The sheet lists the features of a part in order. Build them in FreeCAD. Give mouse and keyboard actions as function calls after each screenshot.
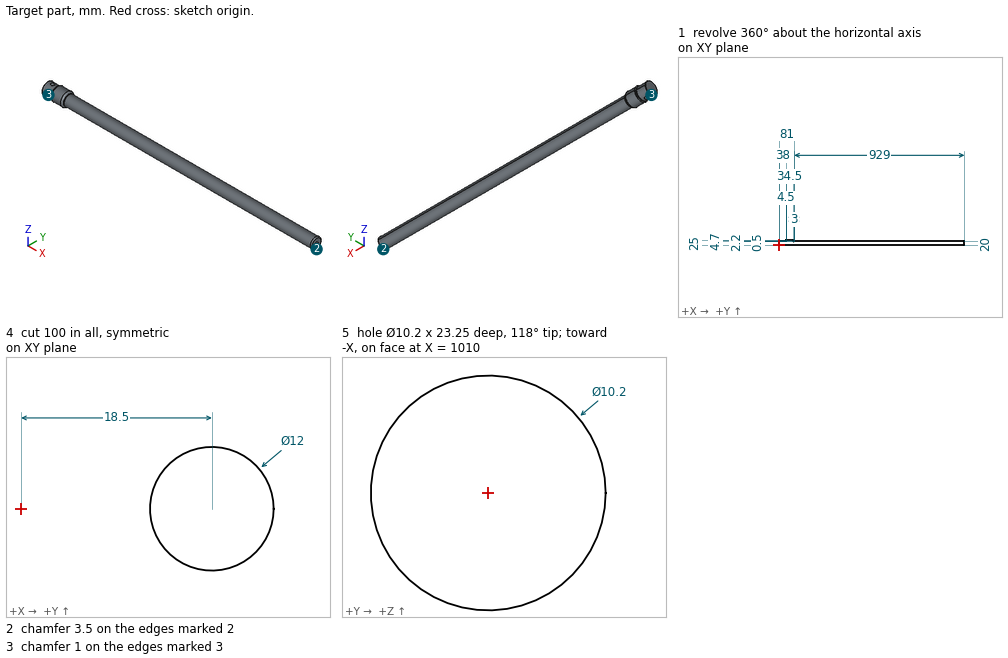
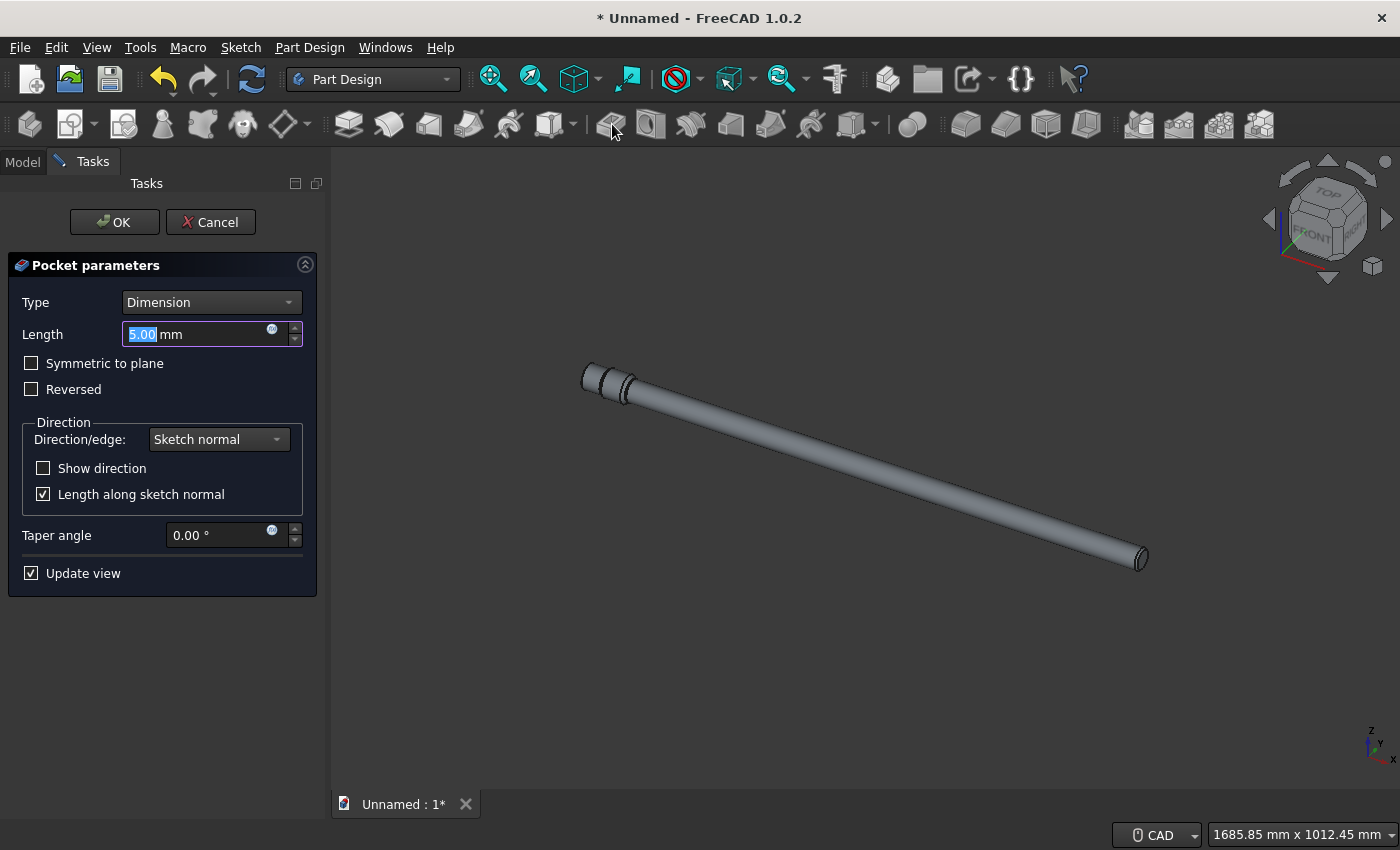
text(100)
key(Tab)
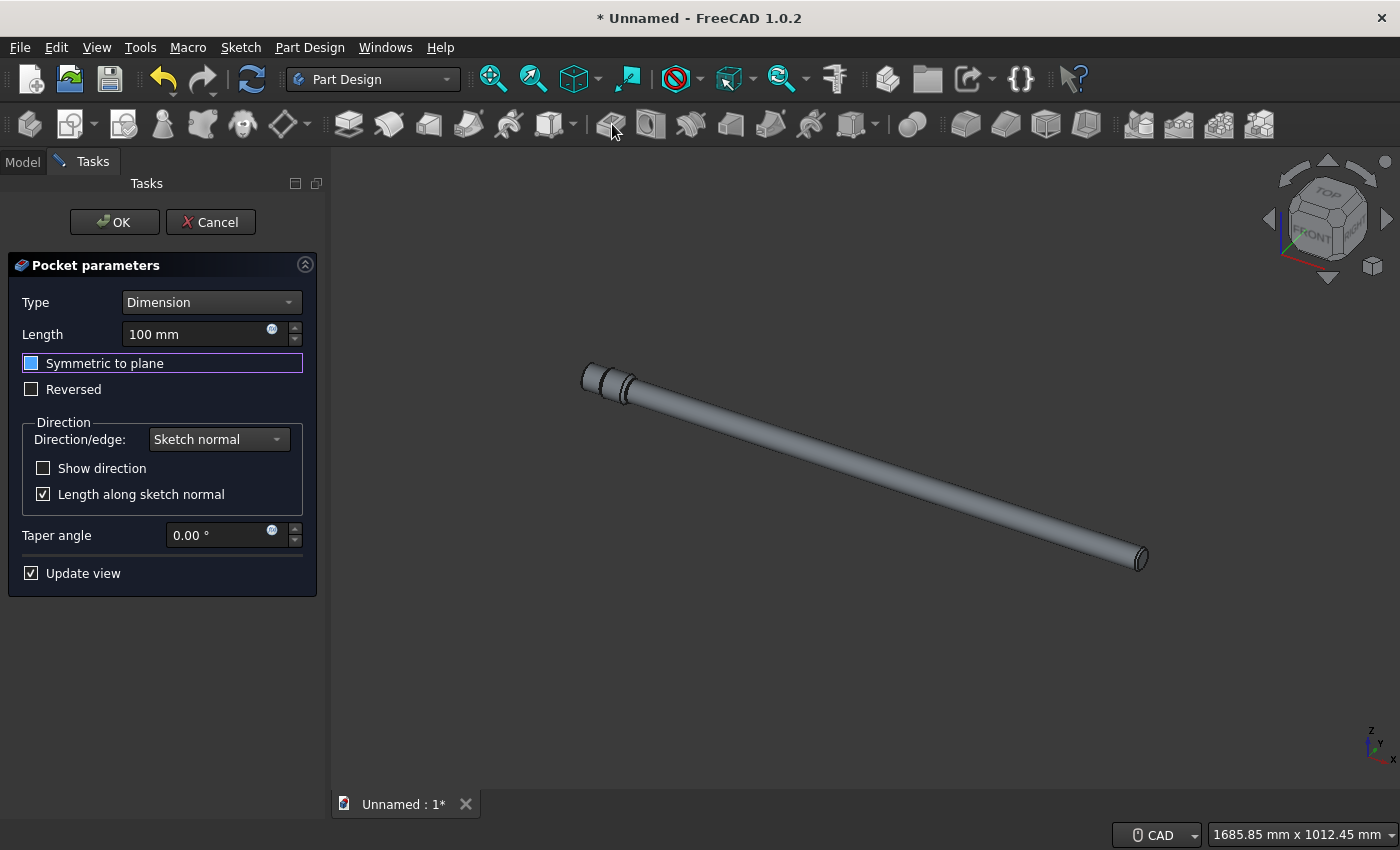
click(30, 363)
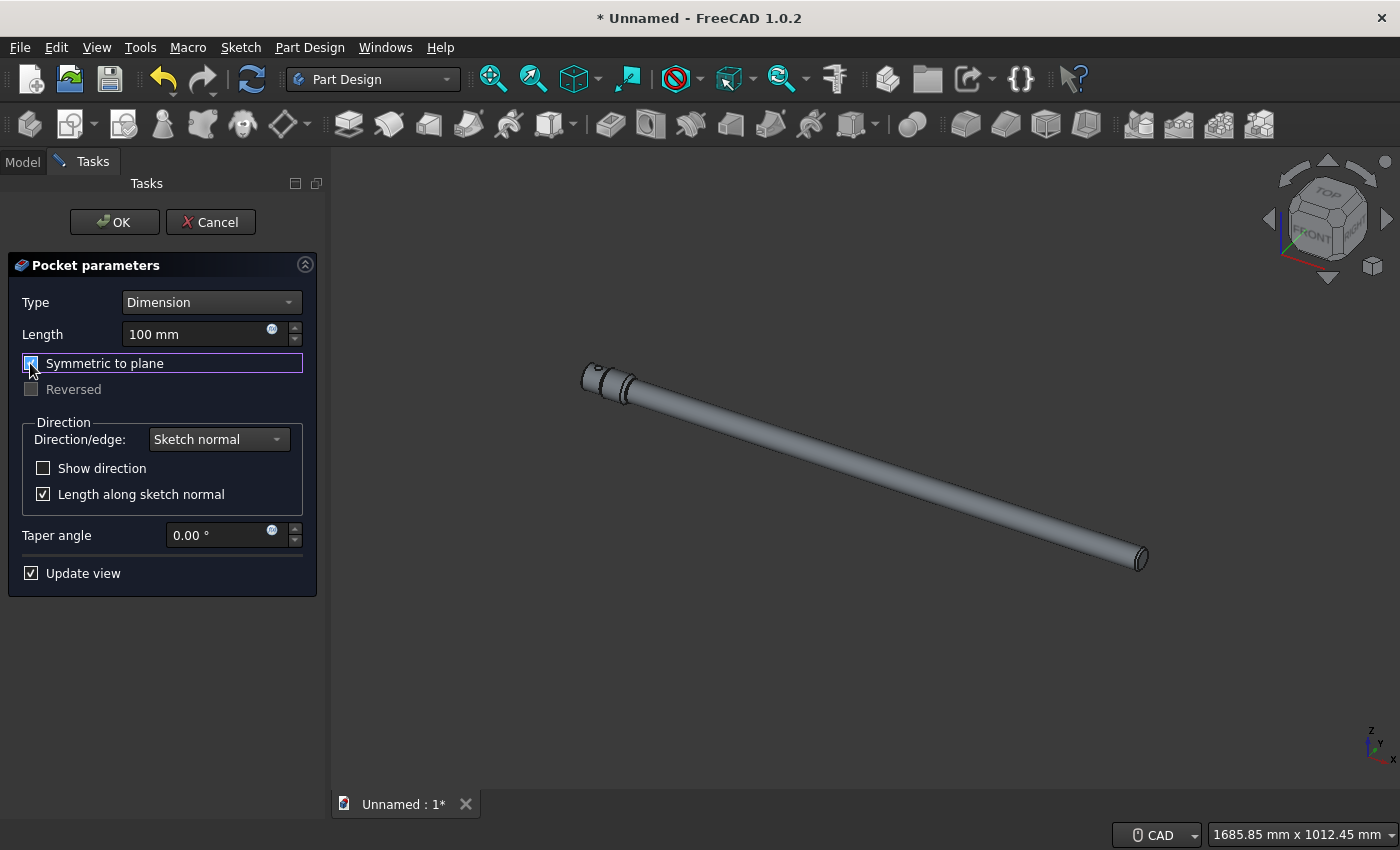
click(115, 222)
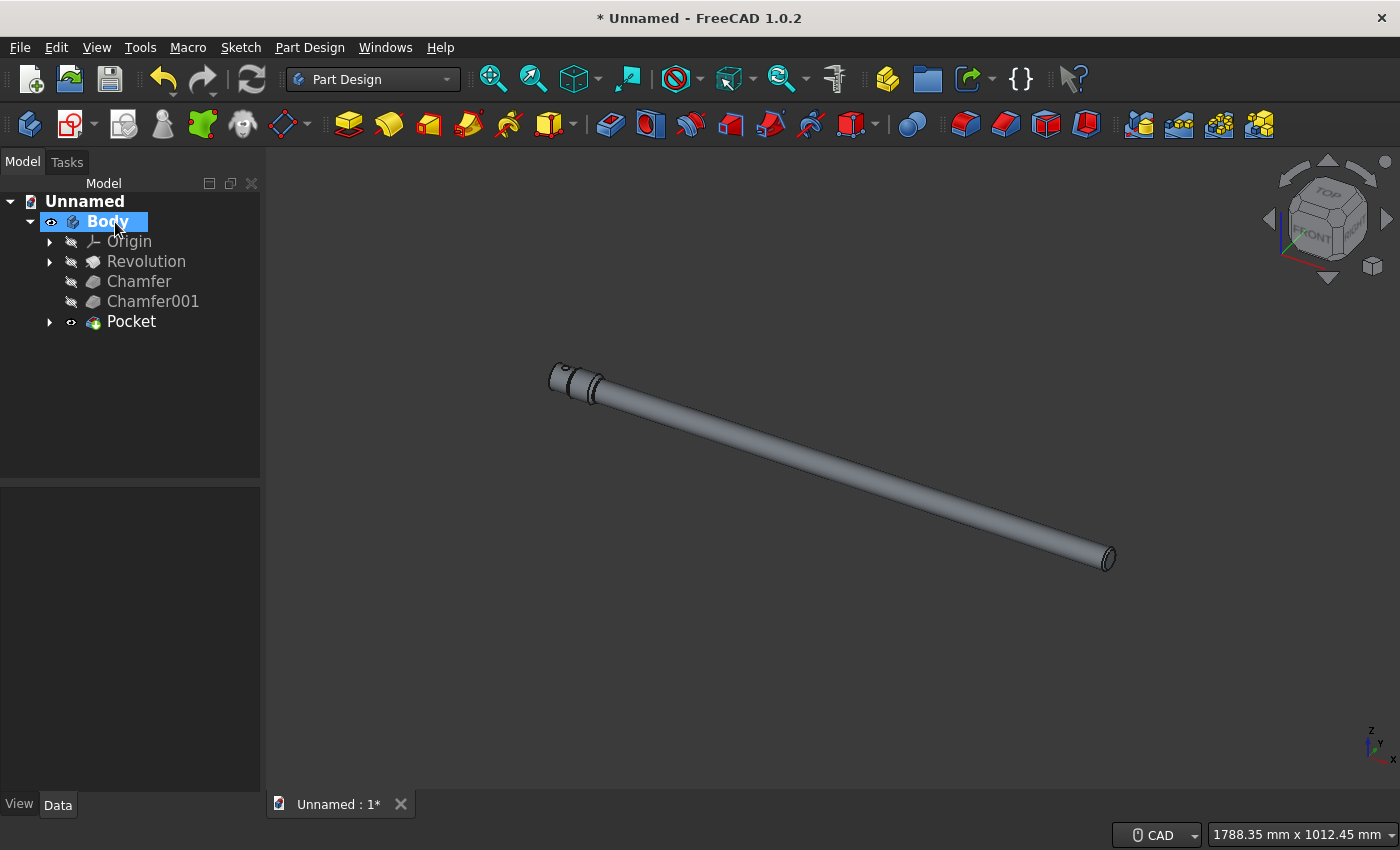
key(0)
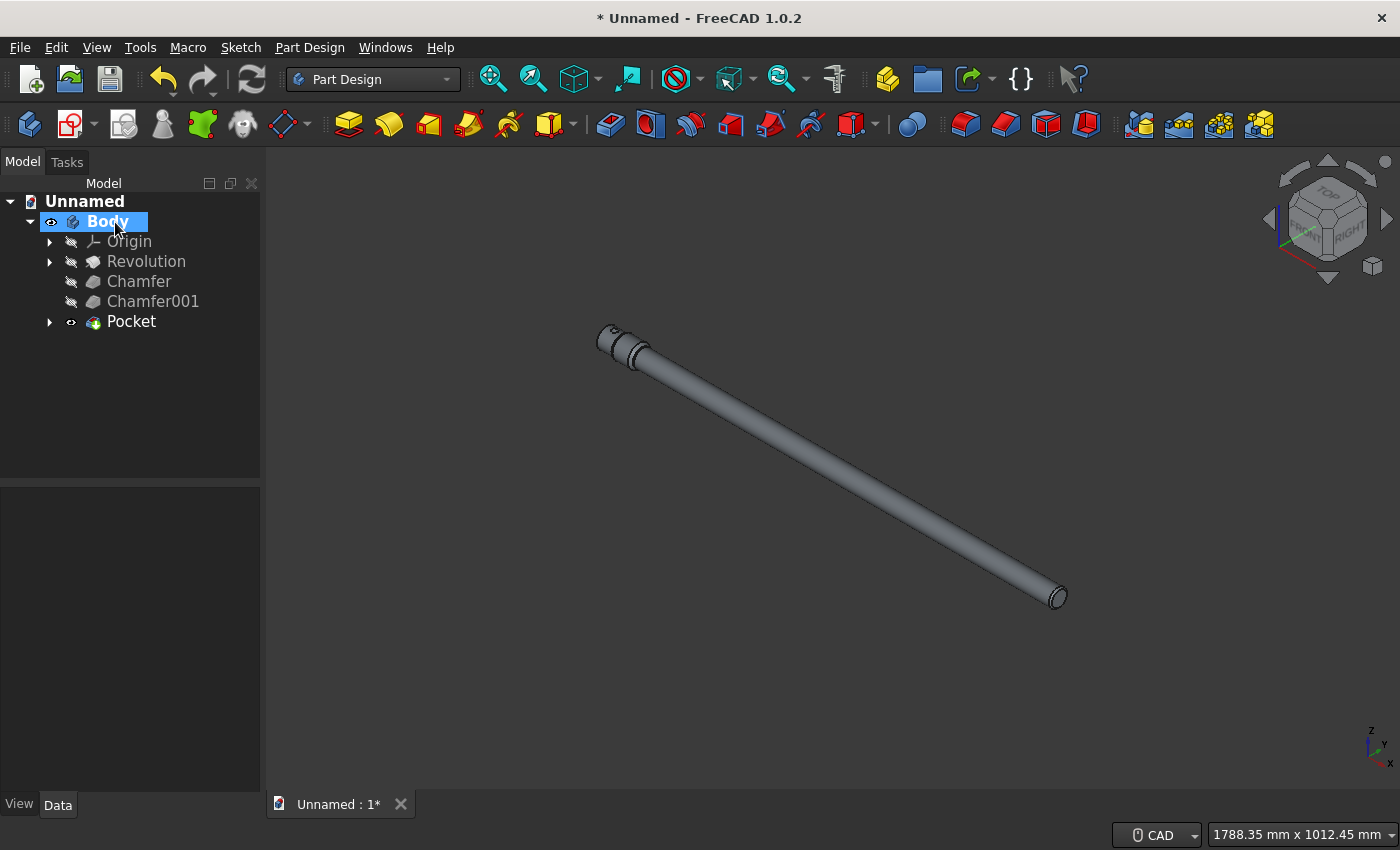
key(3)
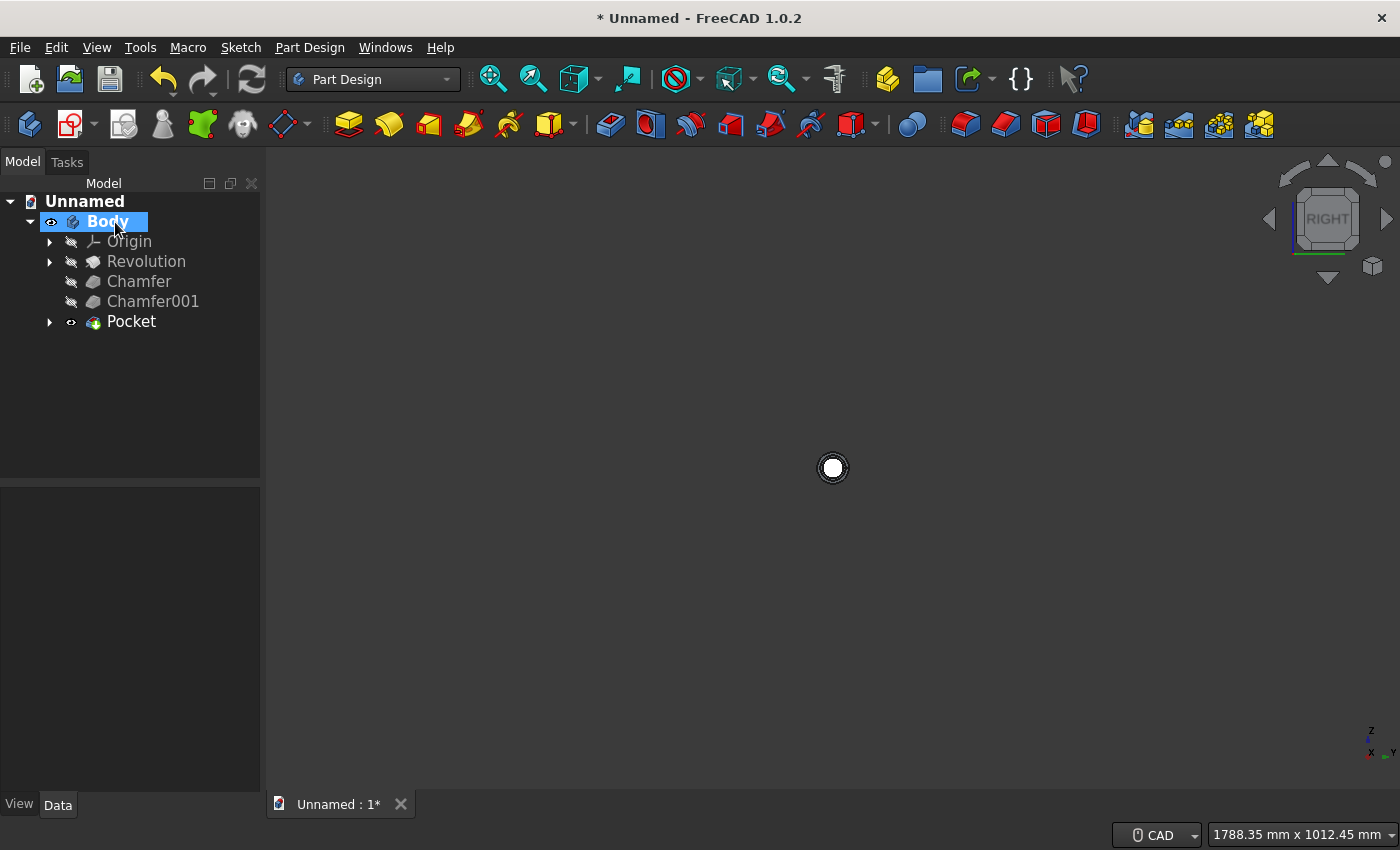
click(494, 80)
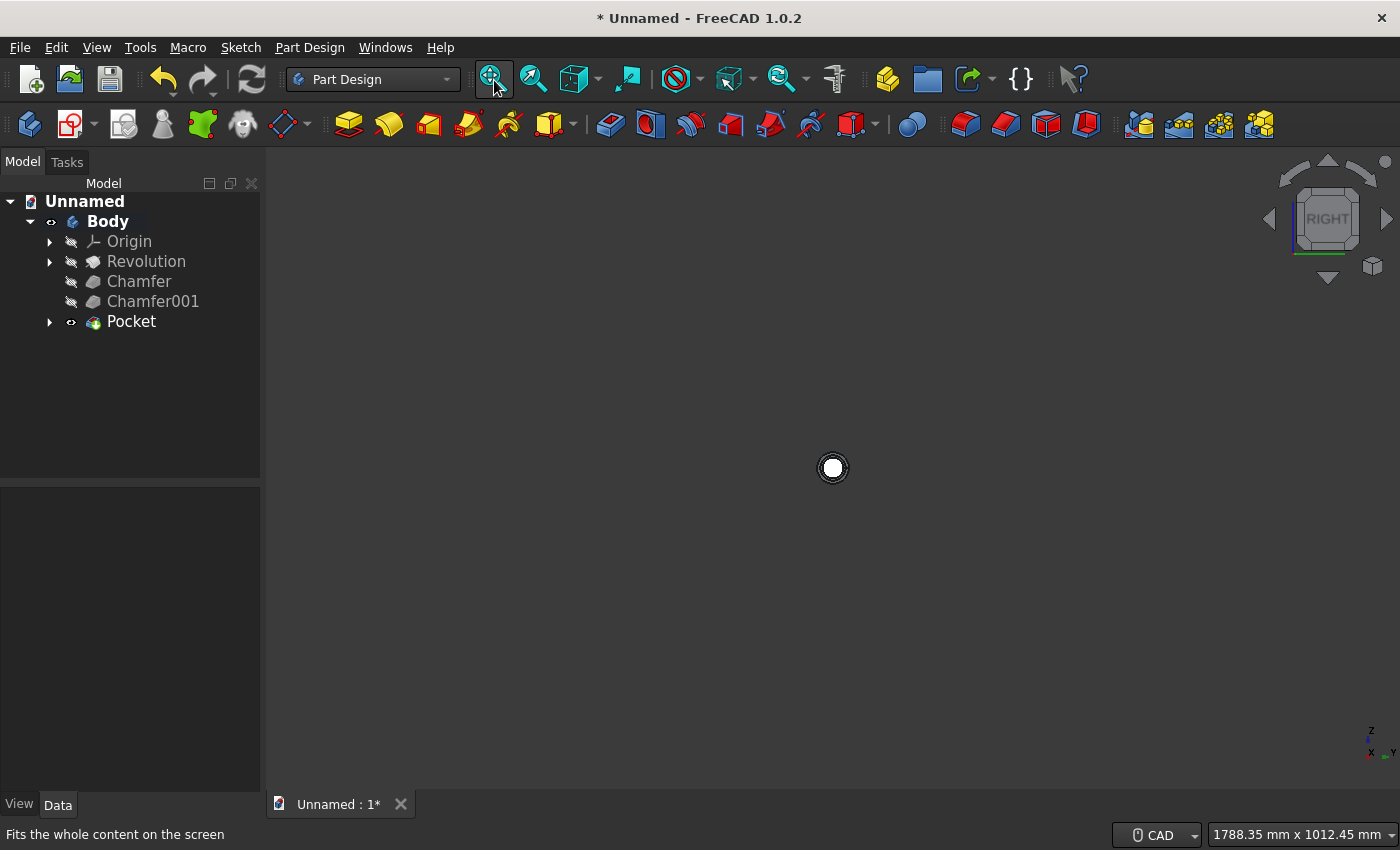
click(833, 467)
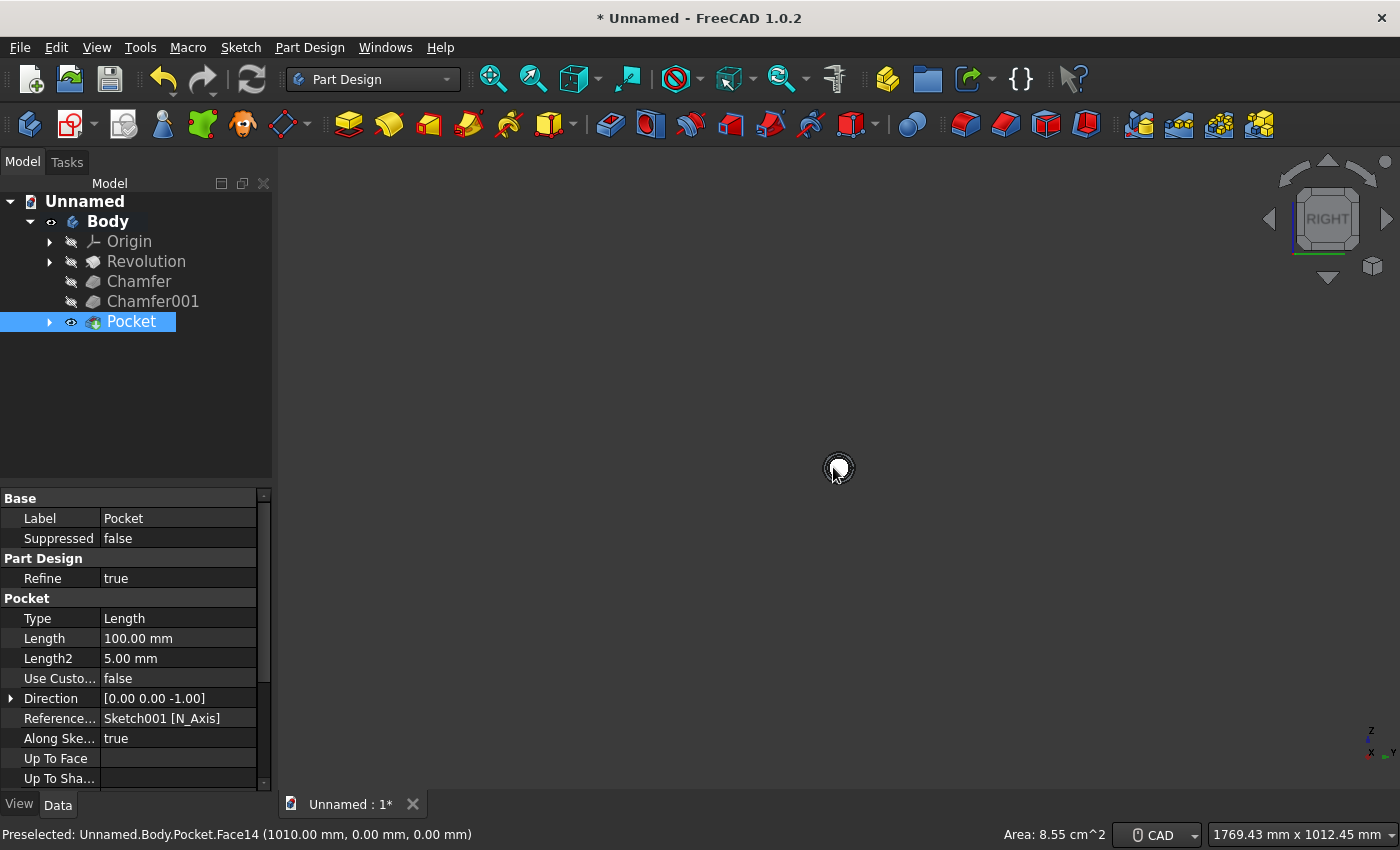
click(70, 124)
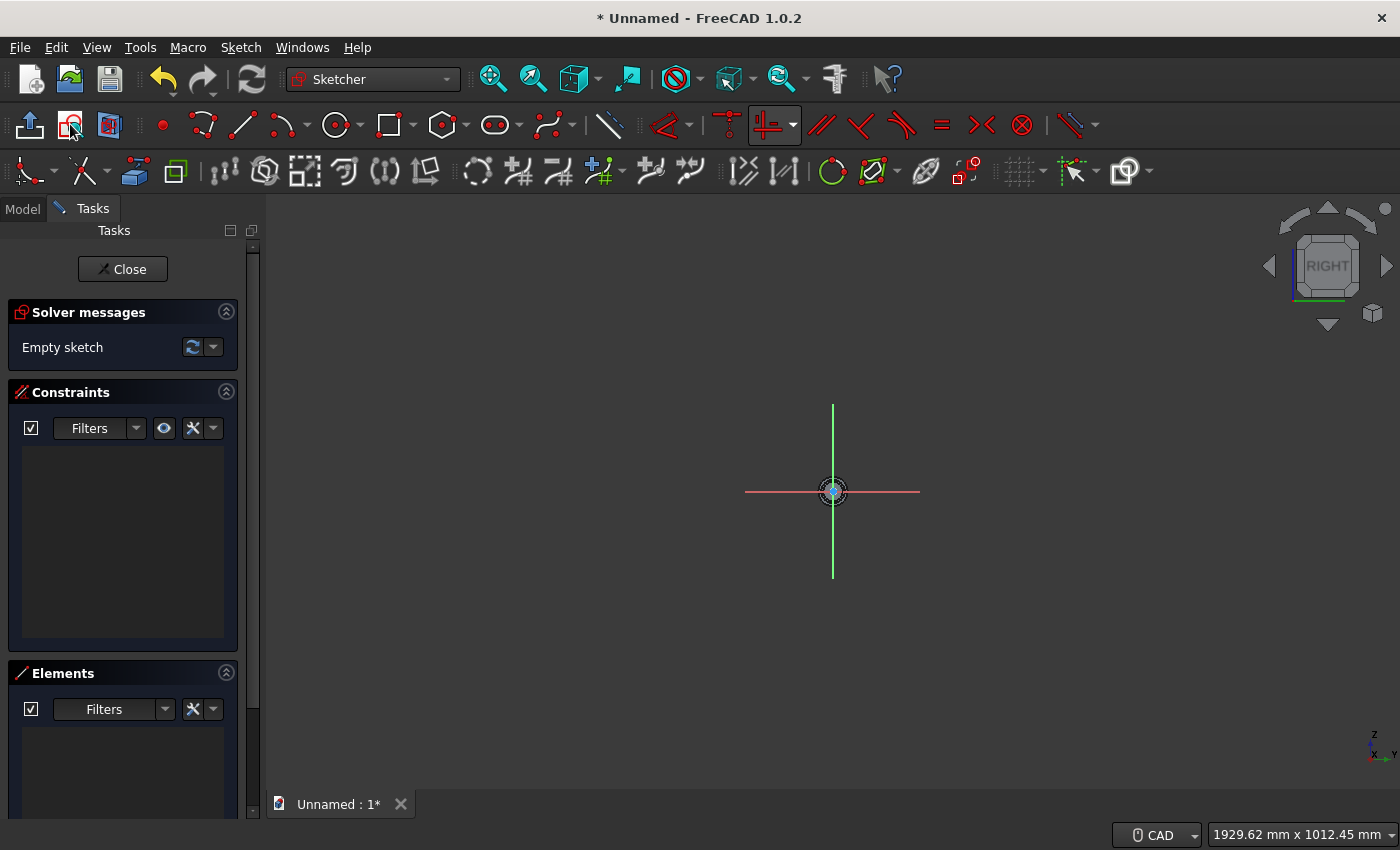
scroll(837, 492, up, 15)